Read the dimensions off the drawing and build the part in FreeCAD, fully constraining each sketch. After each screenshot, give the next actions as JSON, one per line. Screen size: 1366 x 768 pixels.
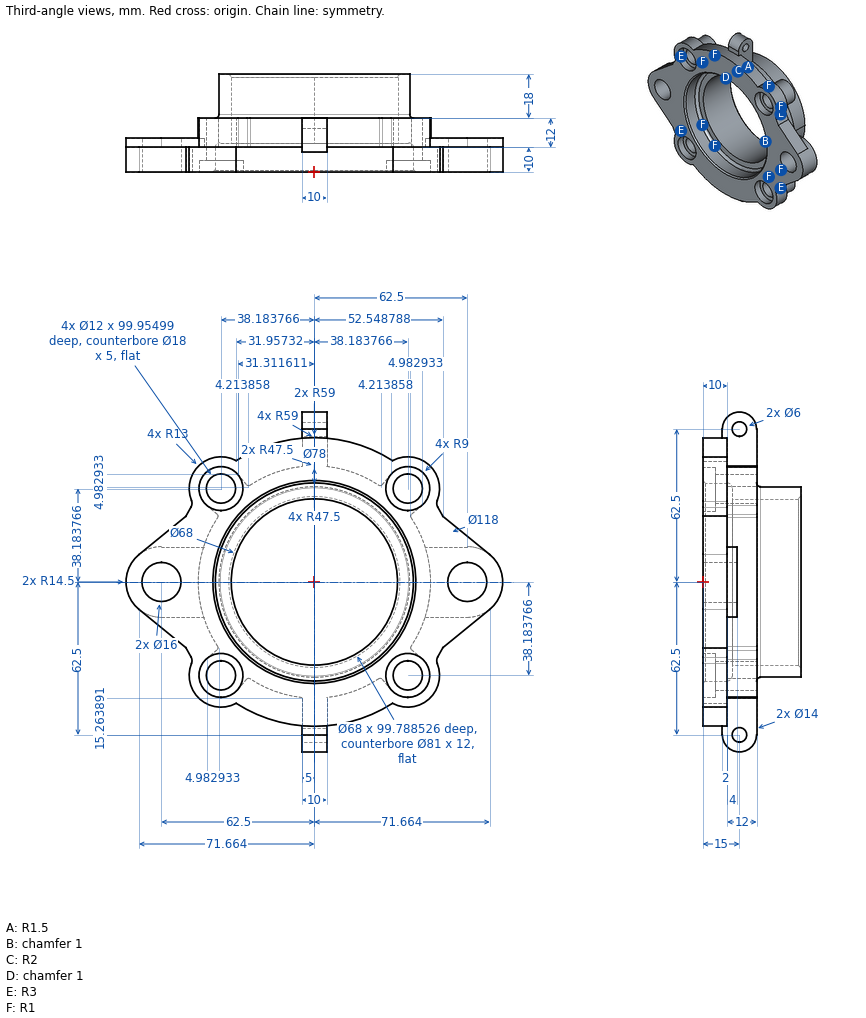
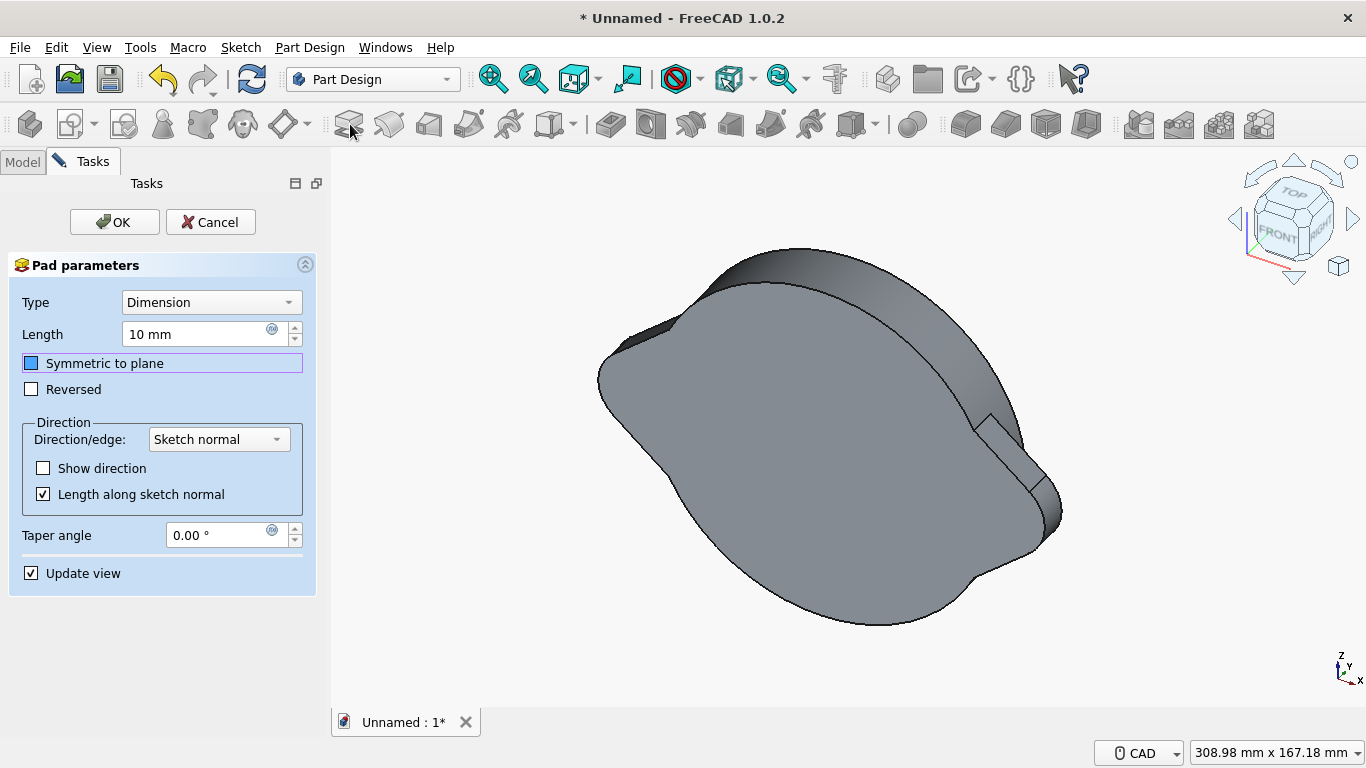
{"action": "left_click", "coordinate": [30, 389]}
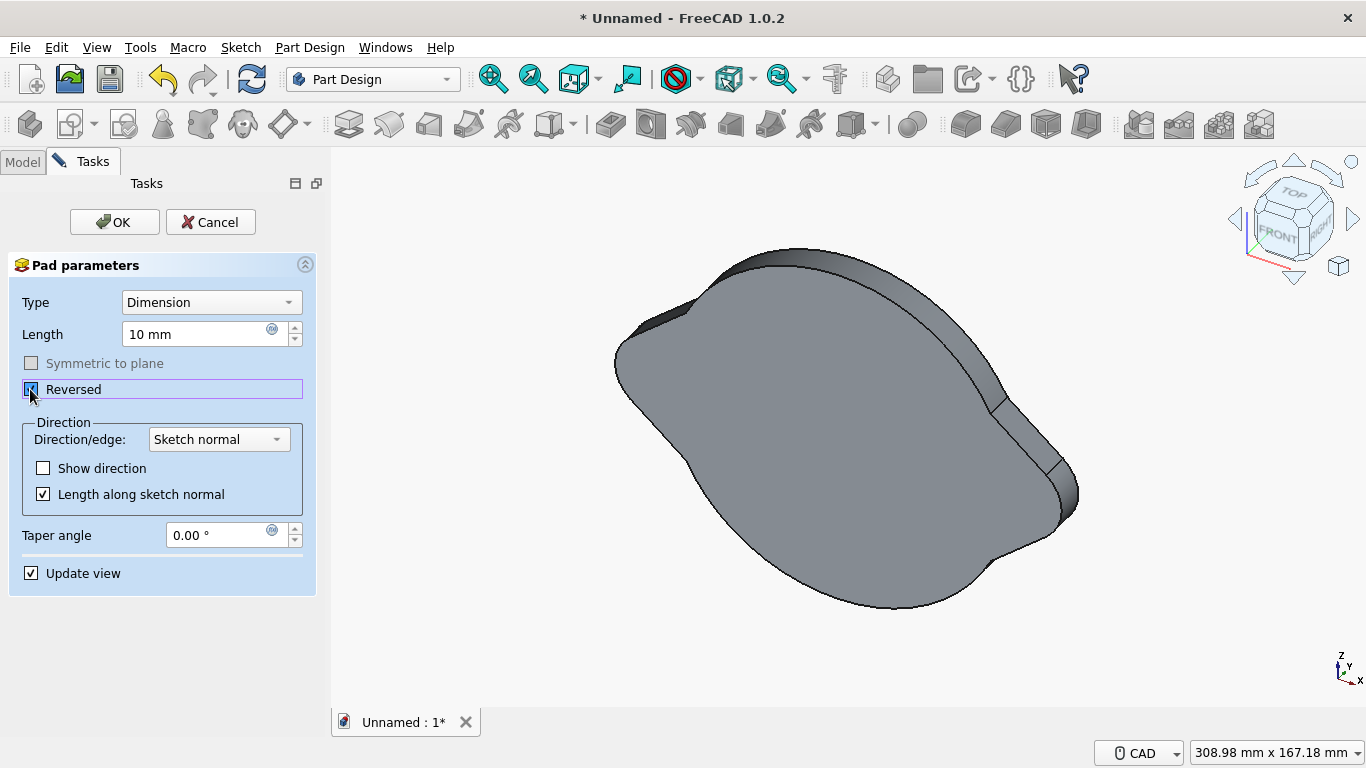
{"action": "left_click", "coordinate": [115, 222]}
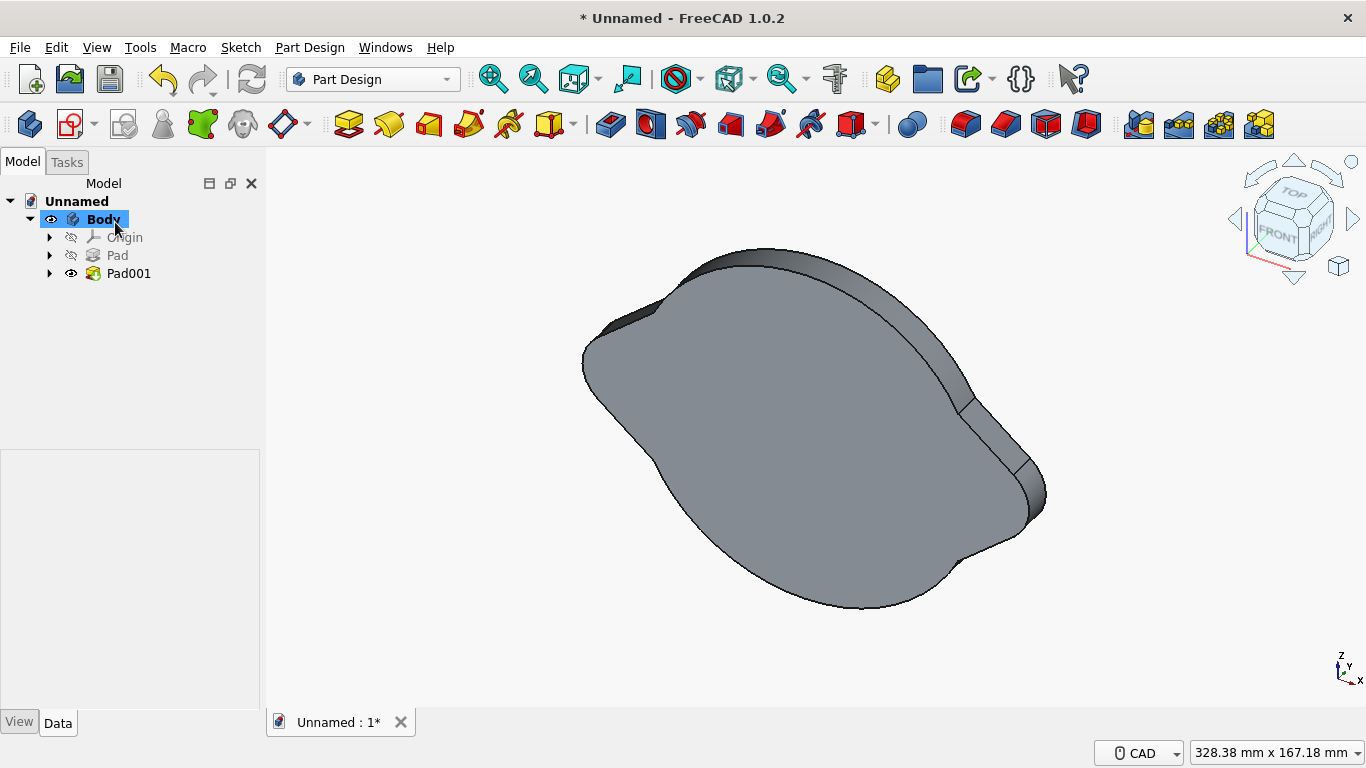
{"action": "left_click", "coordinate": [806, 436]}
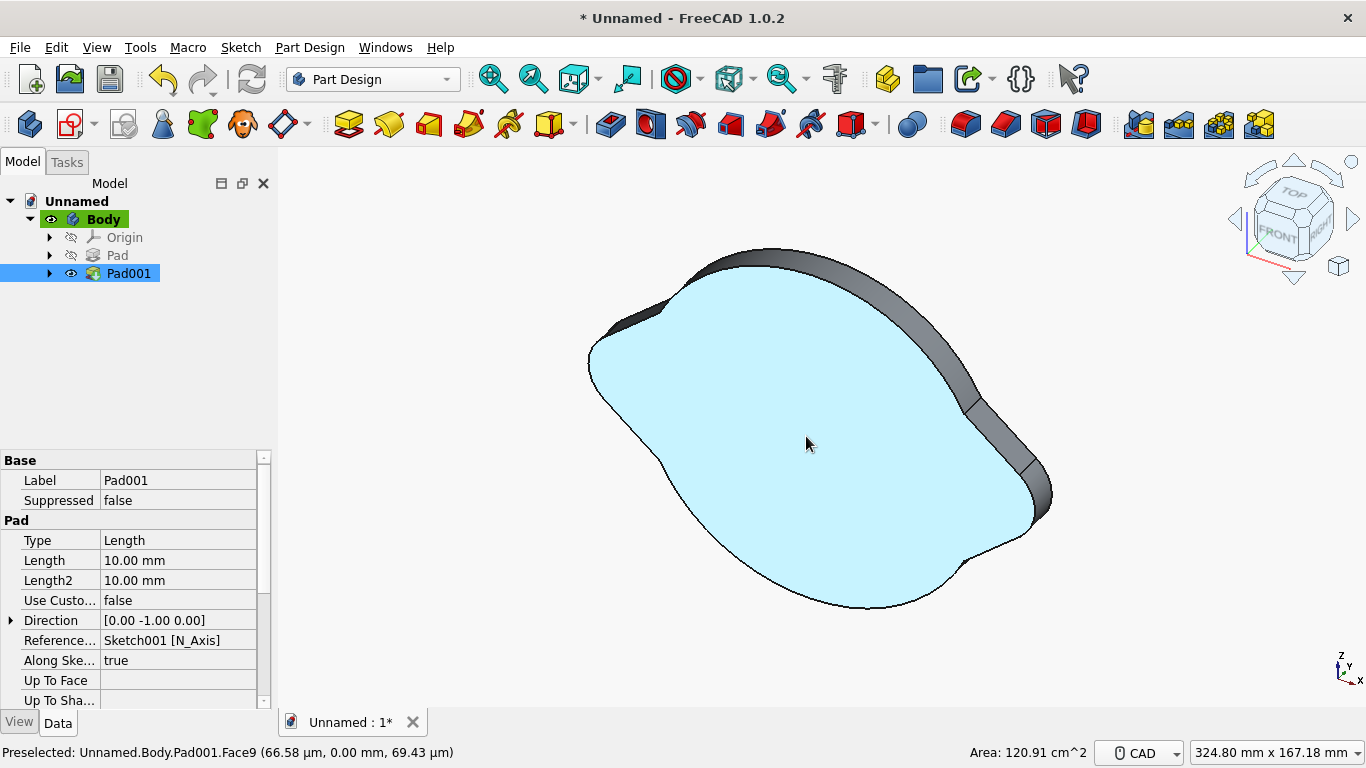
{"action": "left_click", "coordinate": [70, 124]}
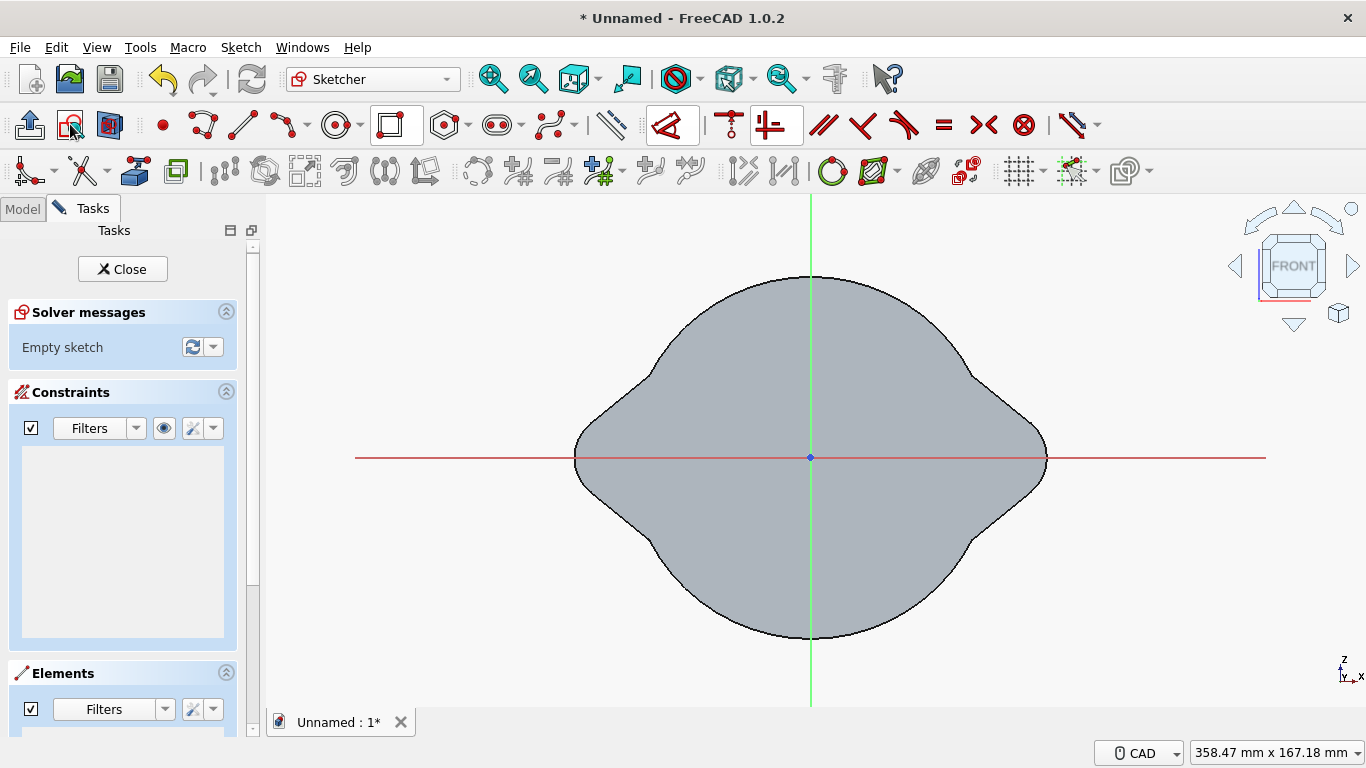
{"action": "left_click", "coordinate": [284, 126]}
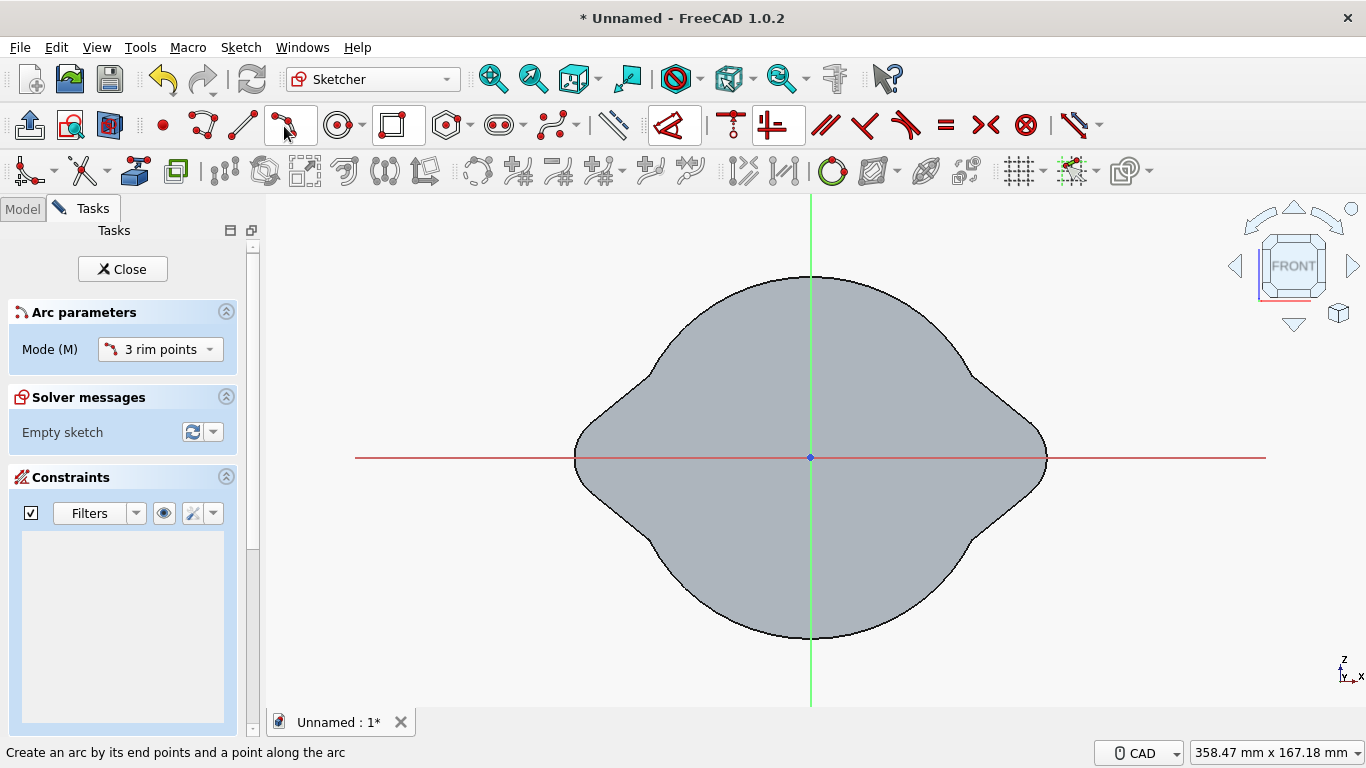
{"action": "left_click", "coordinate": [659, 360]}
{"action": "left_click", "coordinate": [713, 306]}
{"action": "left_click", "coordinate": [665, 313]}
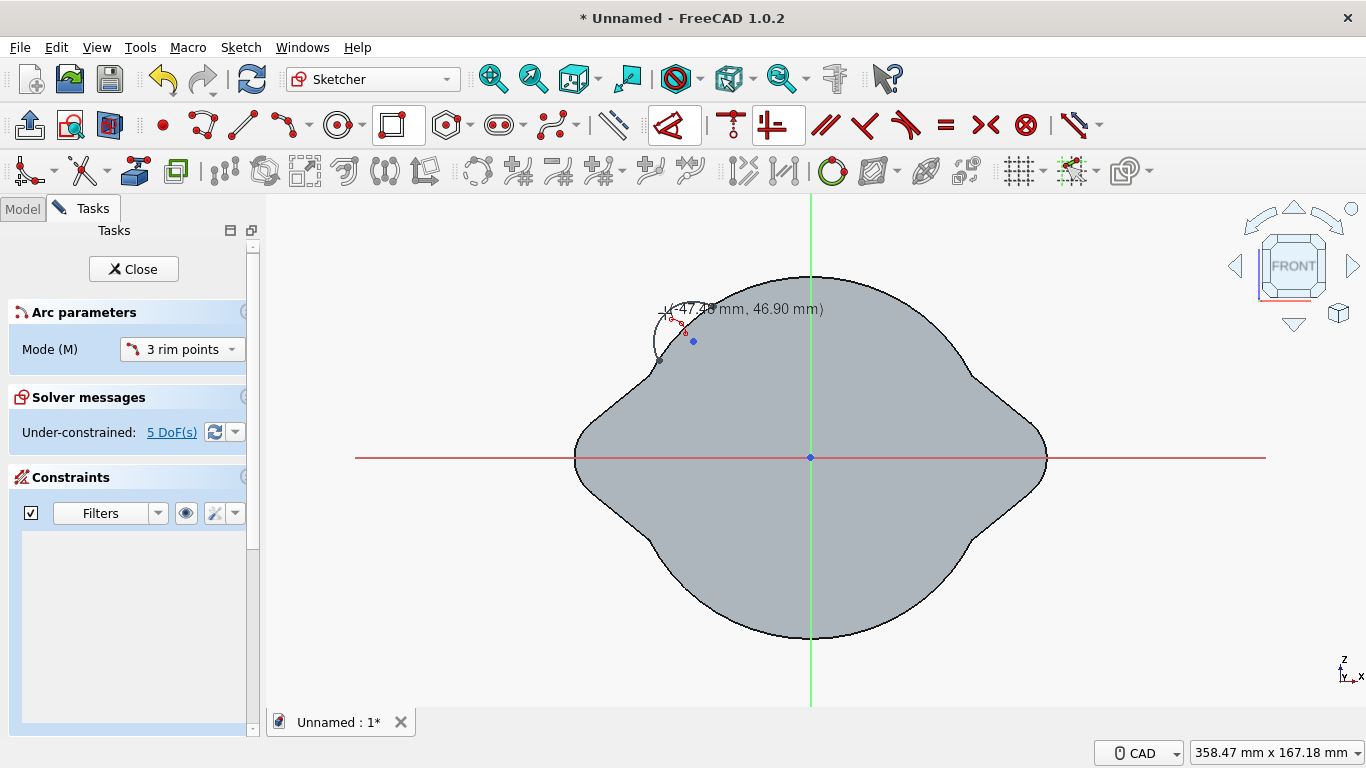
{"action": "left_click", "coordinate": [713, 307]}
{"action": "left_click", "coordinate": [909, 306]}
{"action": "left_click", "coordinate": [831, 278]}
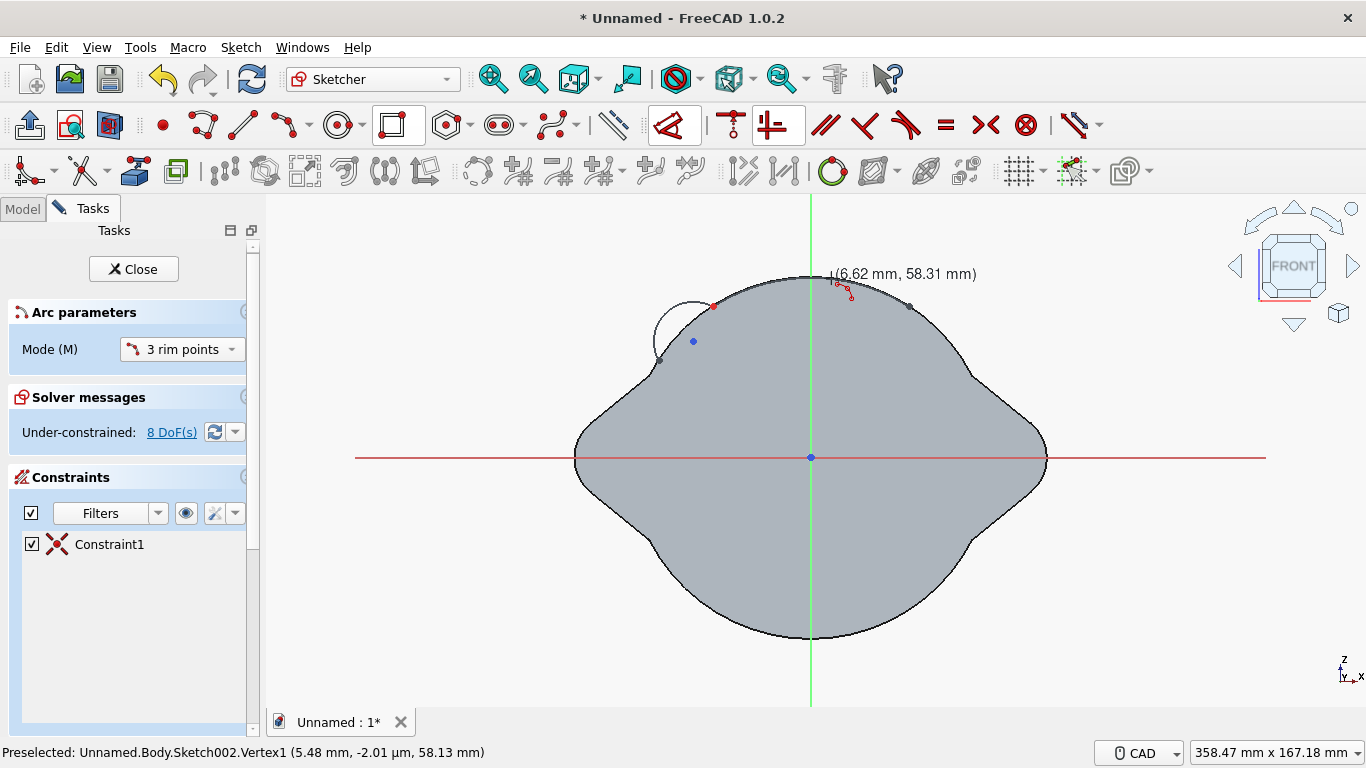
{"action": "left_click", "coordinate": [909, 307]}
{"action": "left_click", "coordinate": [963, 360]}
{"action": "left_click", "coordinate": [956, 313]}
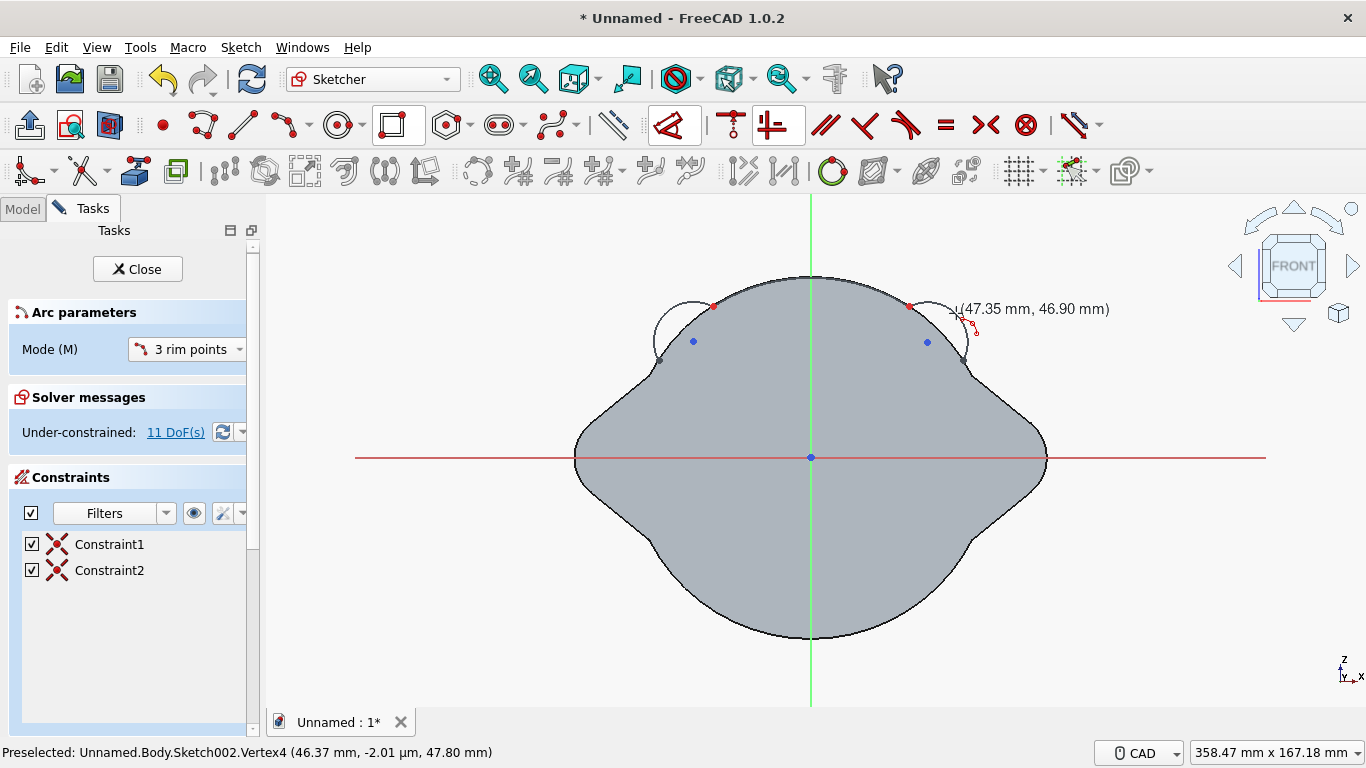
{"action": "left_click", "coordinate": [963, 361]}
{"action": "left_click", "coordinate": [963, 556]}
{"action": "left_click", "coordinate": [991, 479]}